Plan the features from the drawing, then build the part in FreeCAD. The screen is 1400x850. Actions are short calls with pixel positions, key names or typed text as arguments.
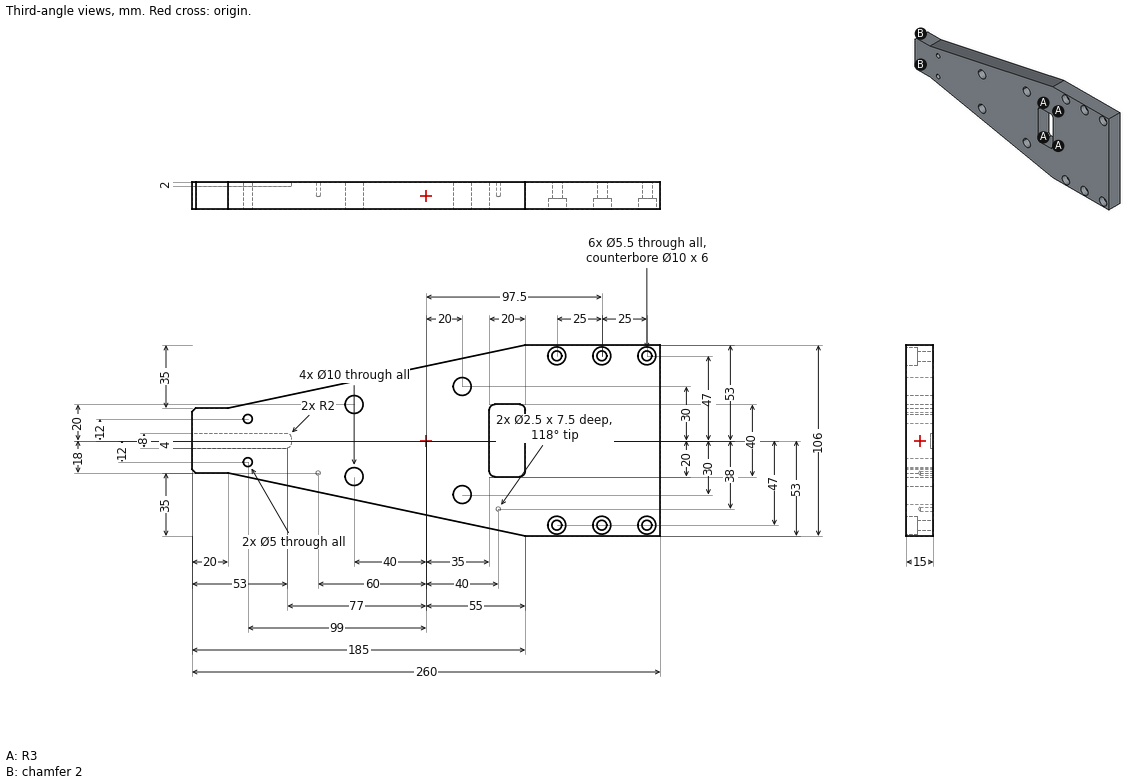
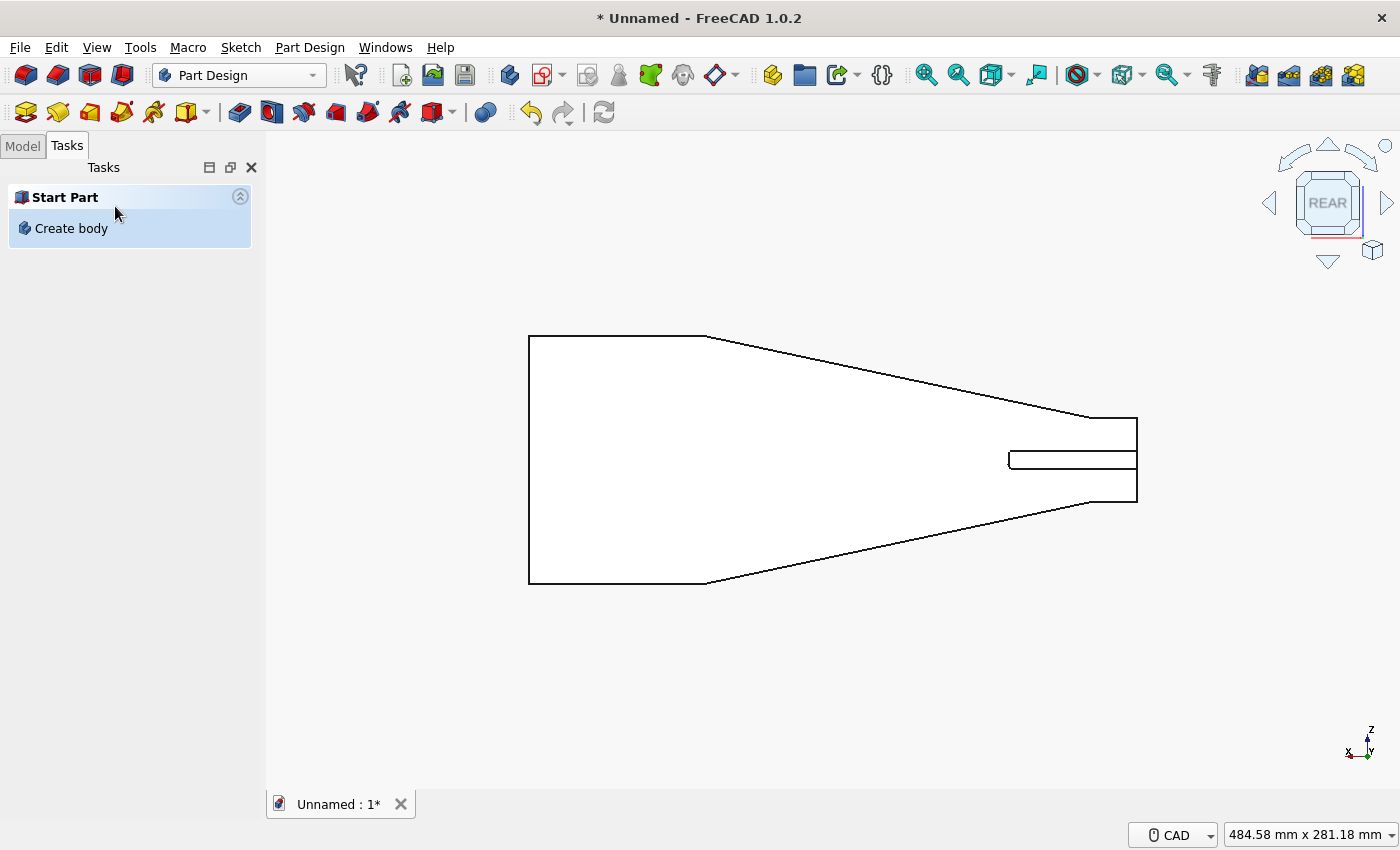
click(659, 459)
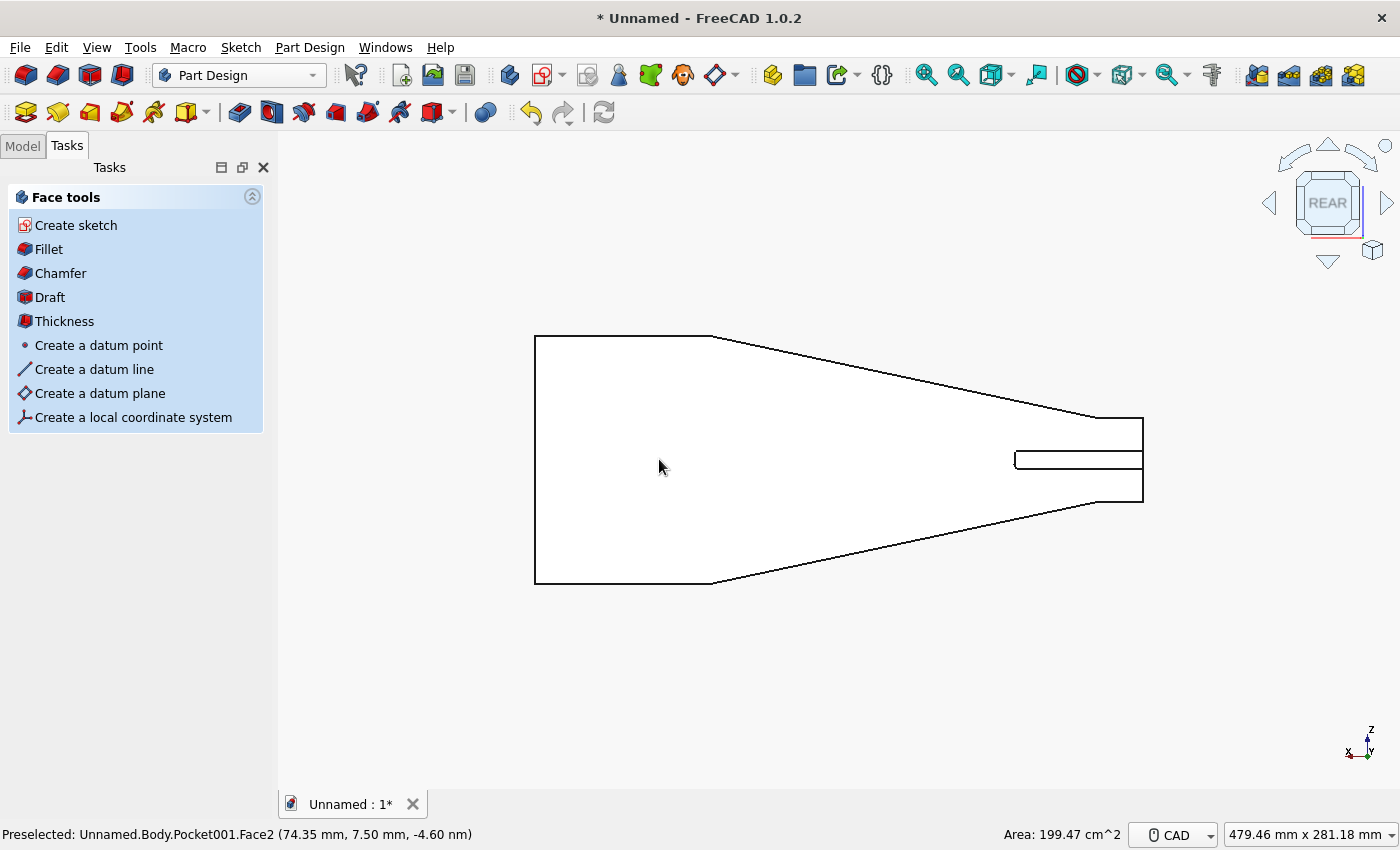
click(542, 76)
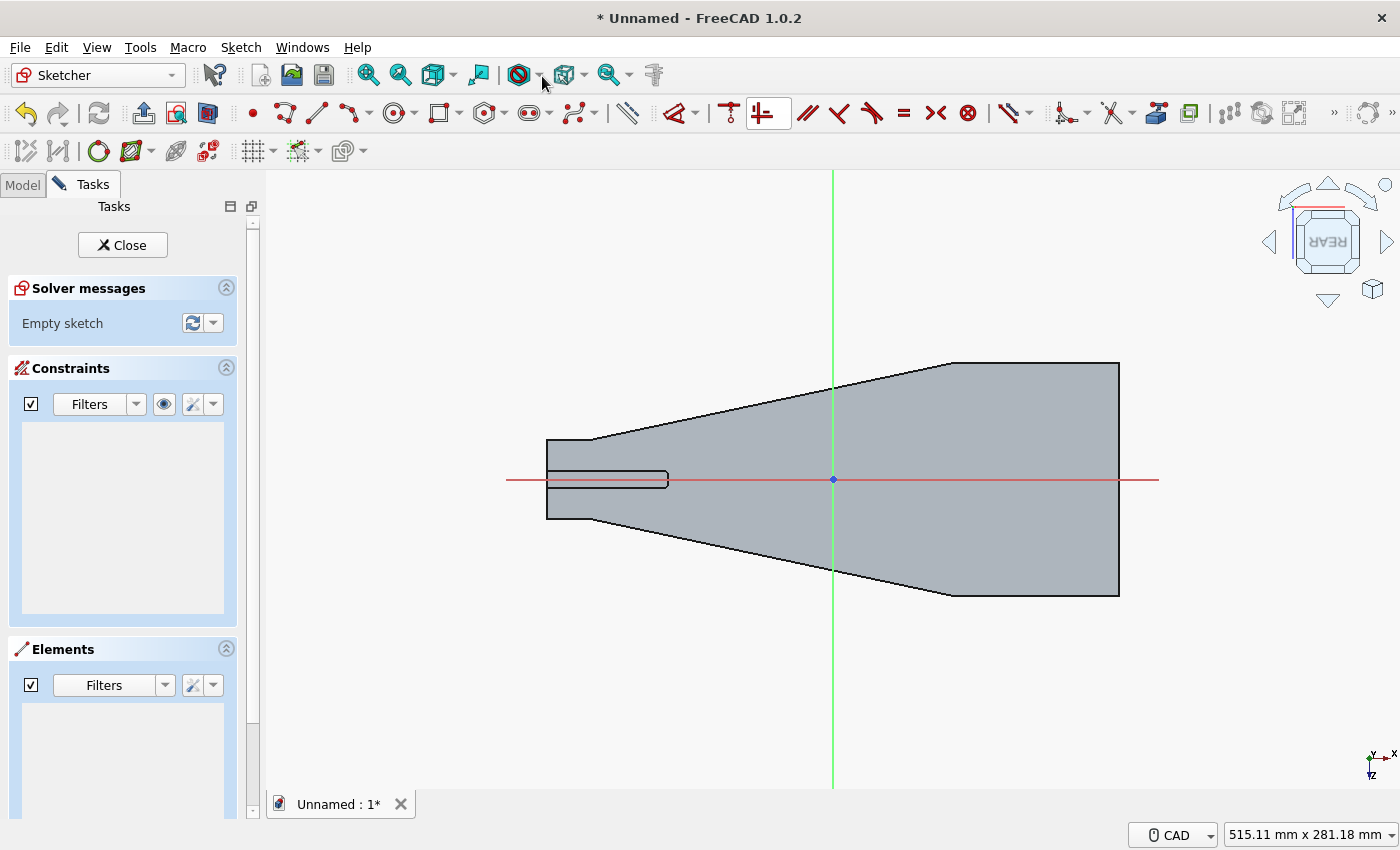
scroll(585, 479, up, 9)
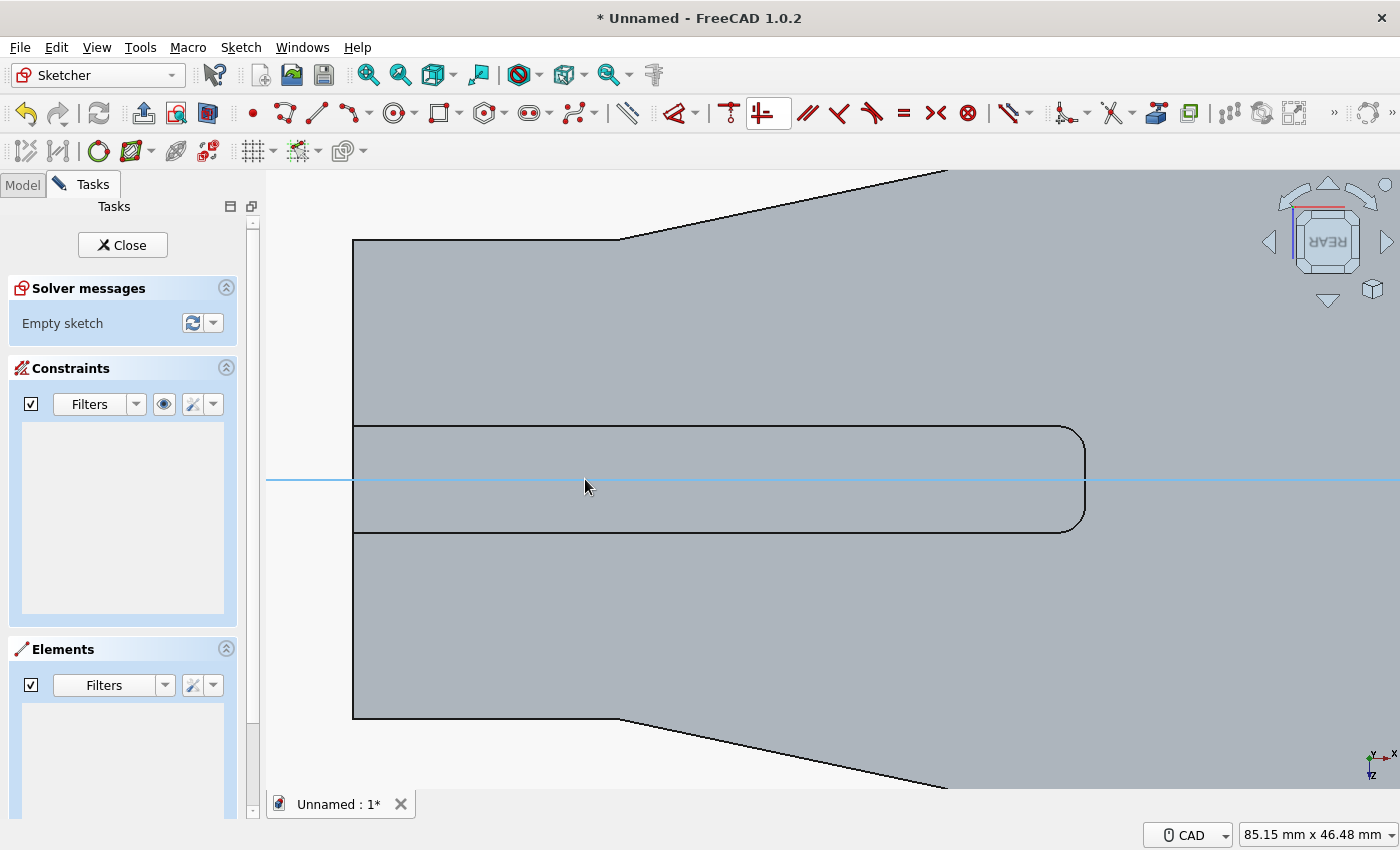
key(g)
key(c)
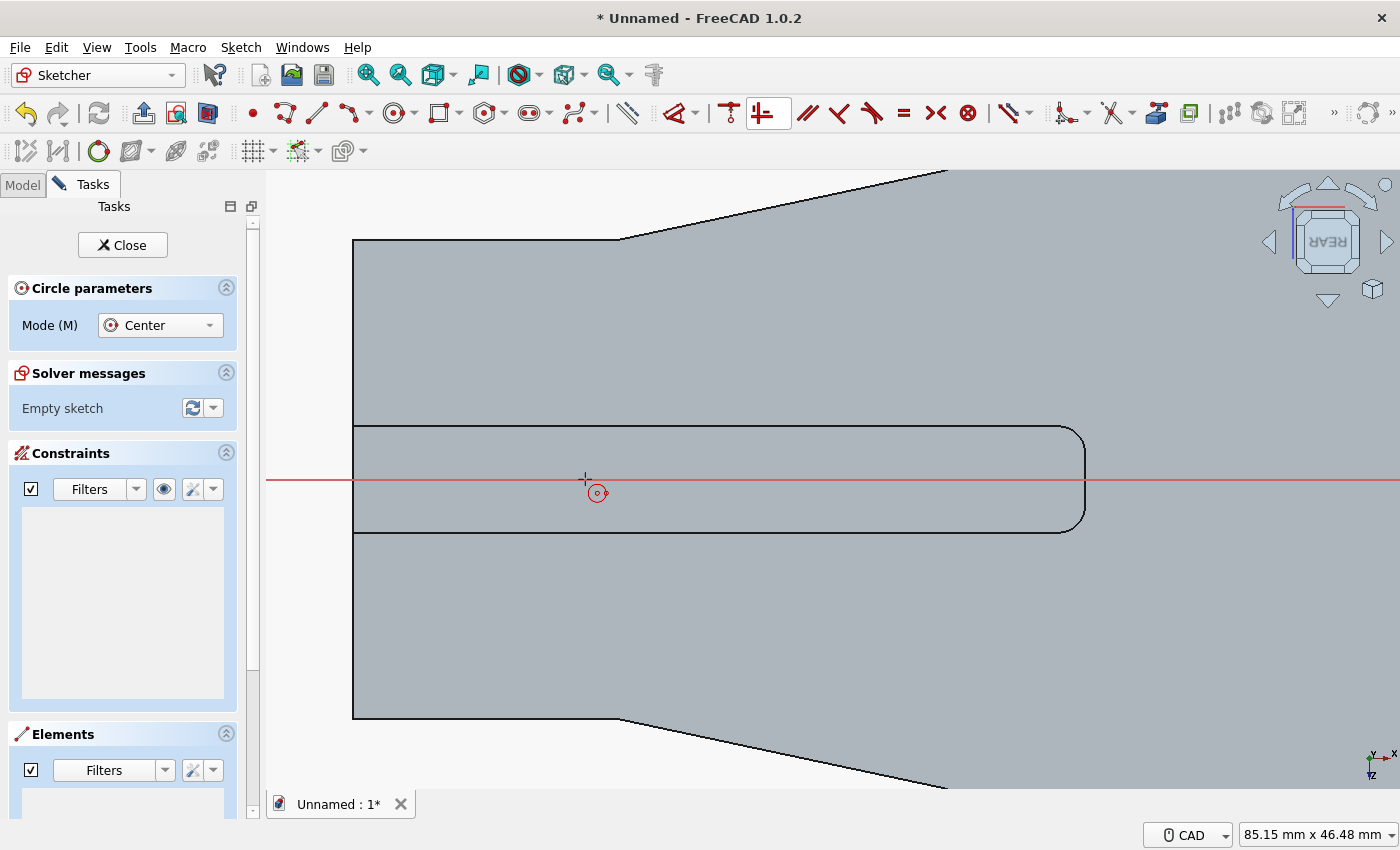
click(765, 320)
click(789, 296)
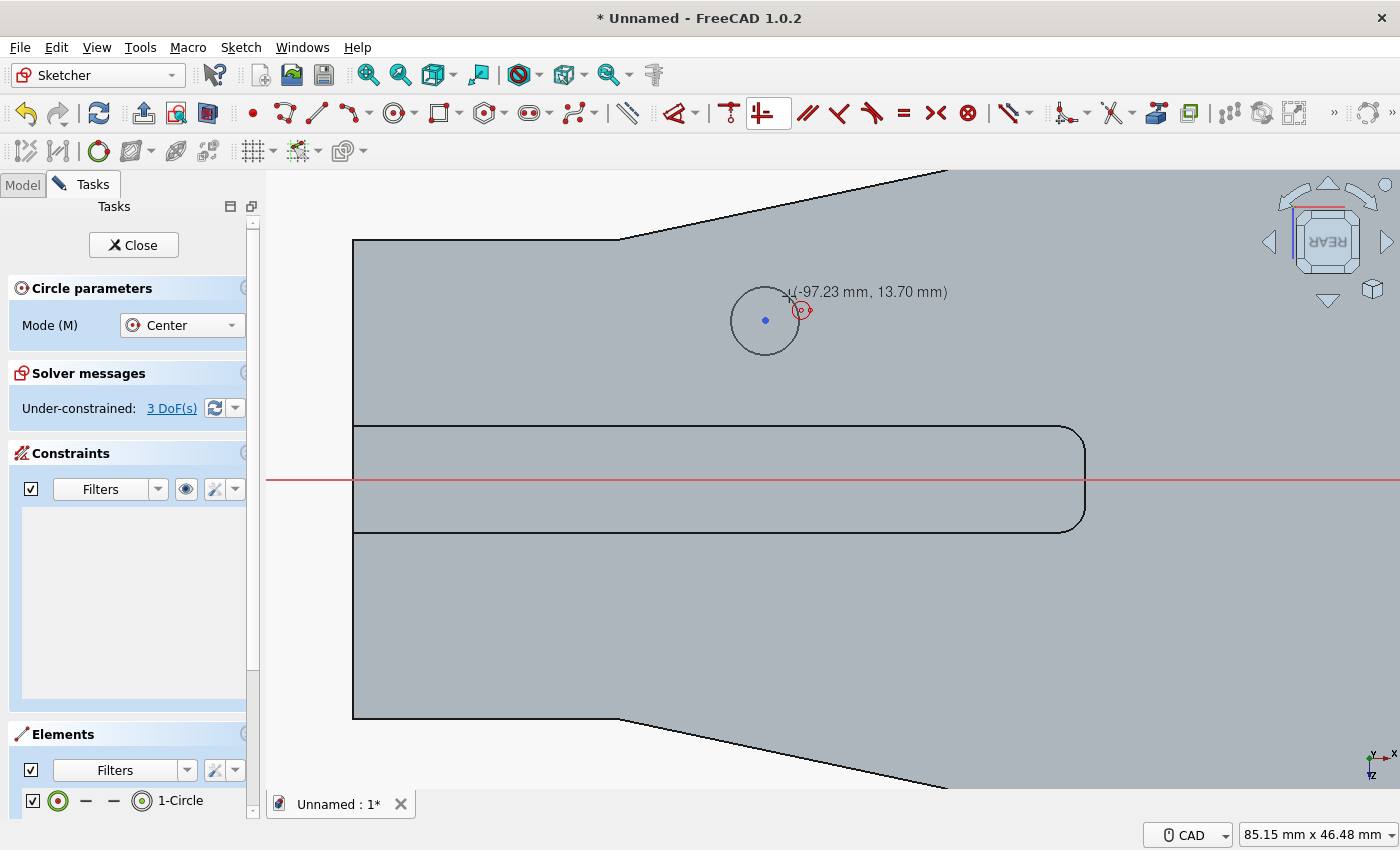
click(765, 639)
click(789, 616)
key(Escape)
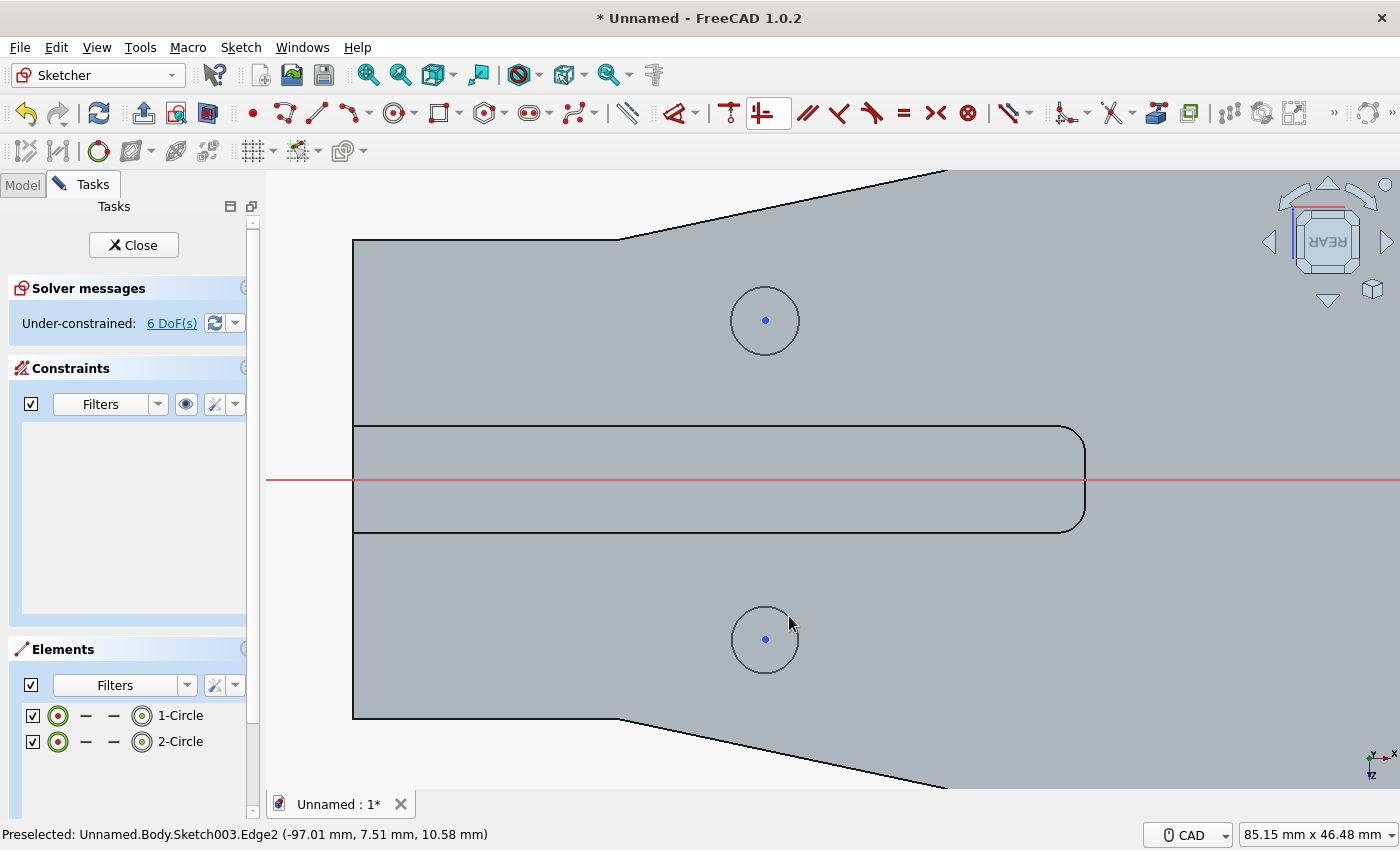
click(789, 297)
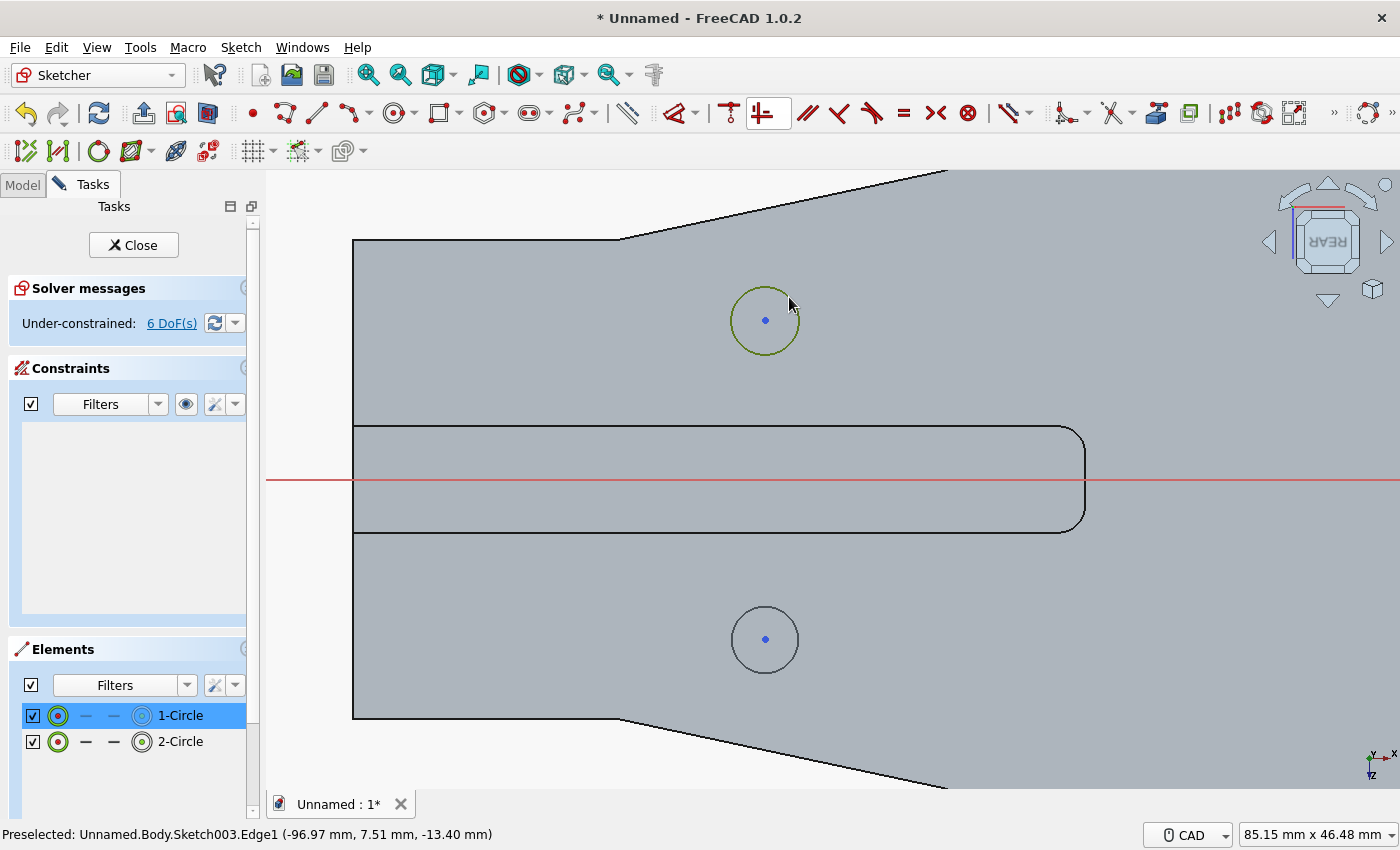
click(788, 616)